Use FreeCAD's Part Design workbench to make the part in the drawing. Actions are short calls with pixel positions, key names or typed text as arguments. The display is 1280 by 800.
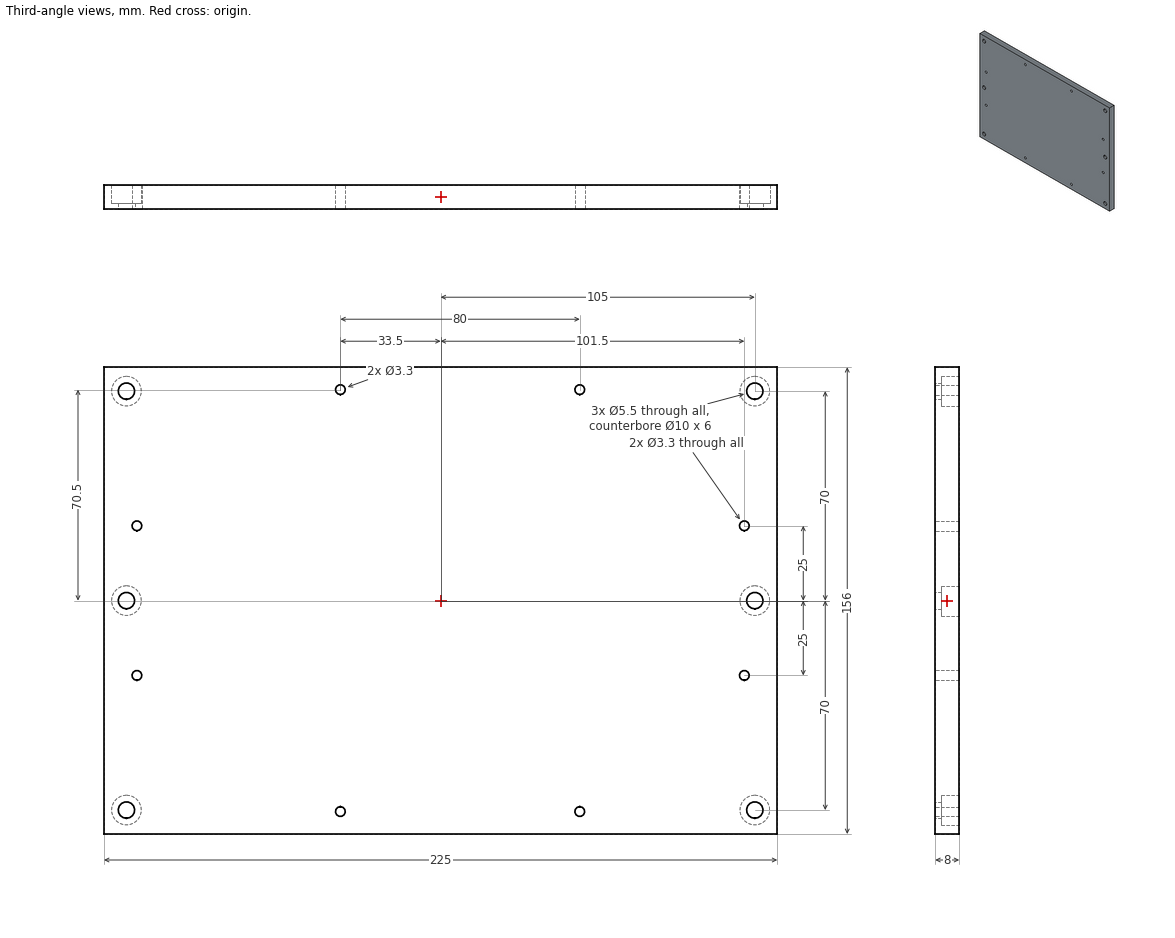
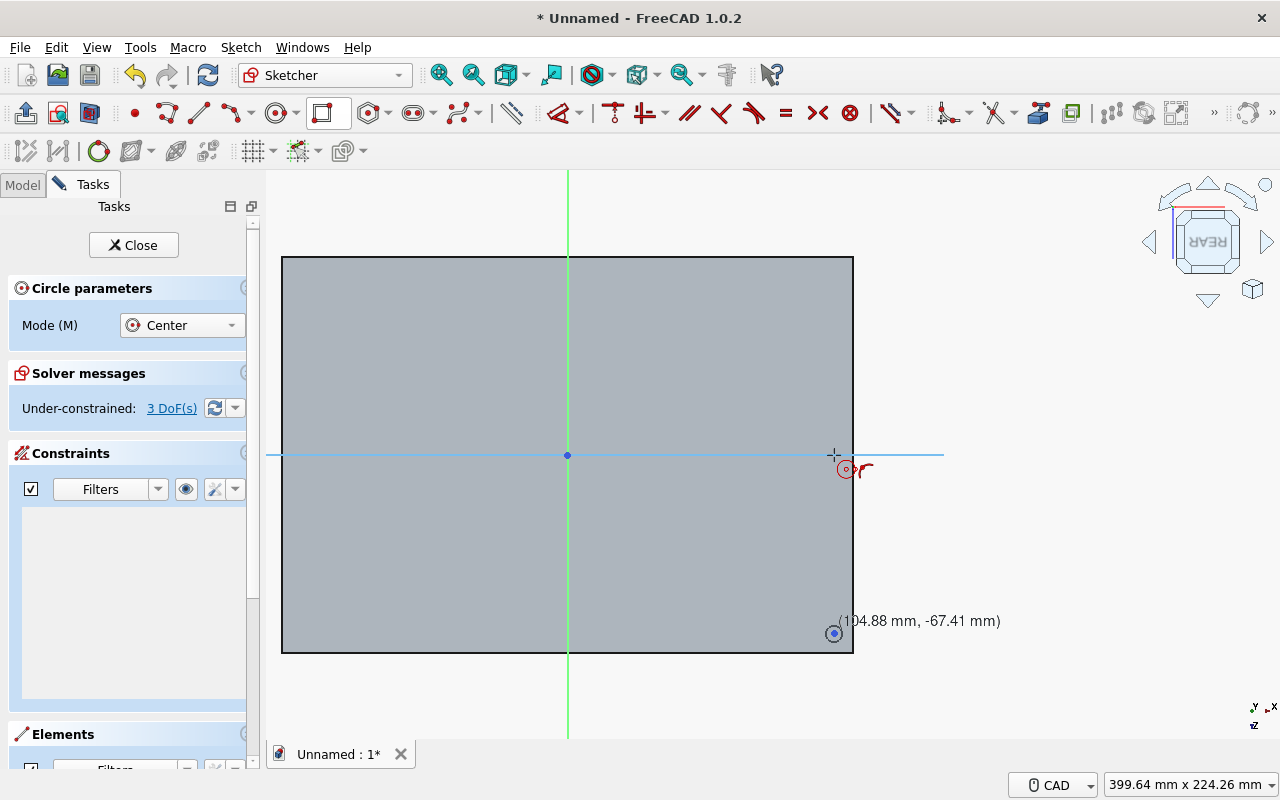
click(834, 455)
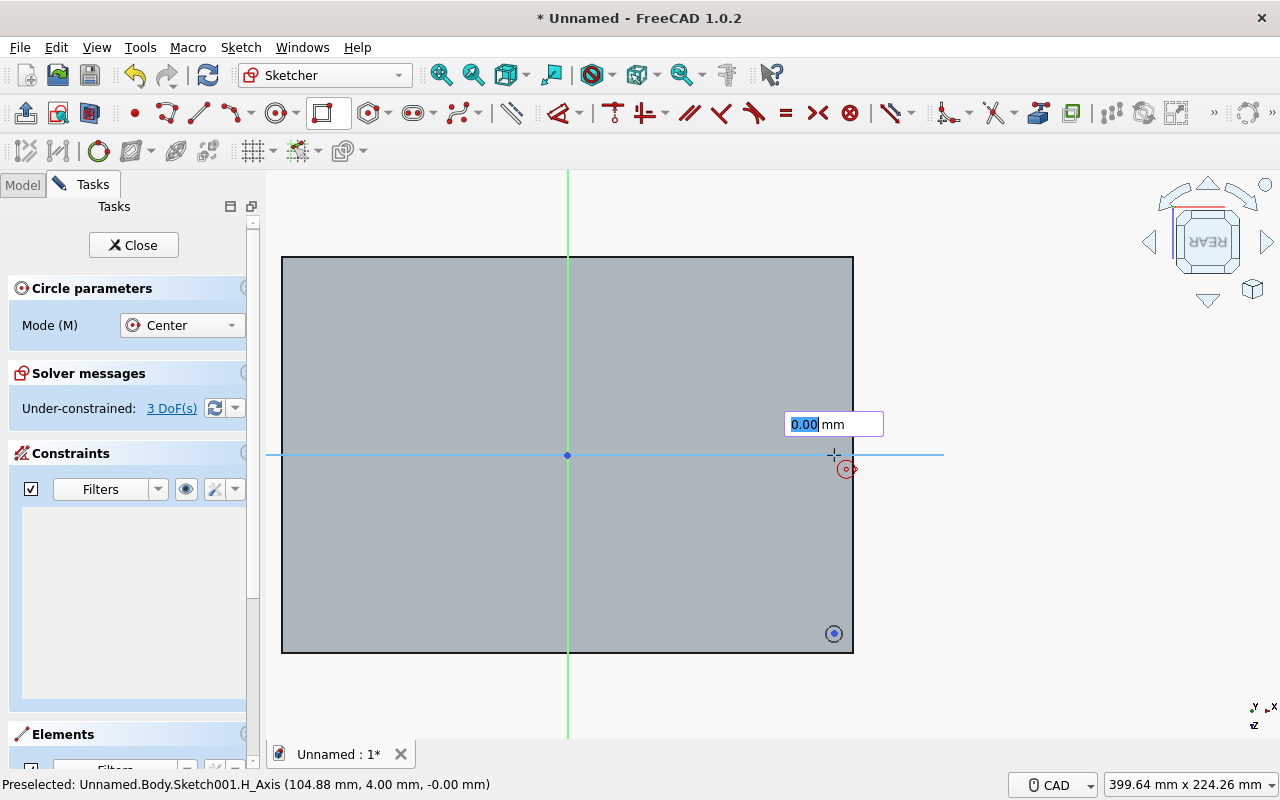
scroll(837, 448, up, 5)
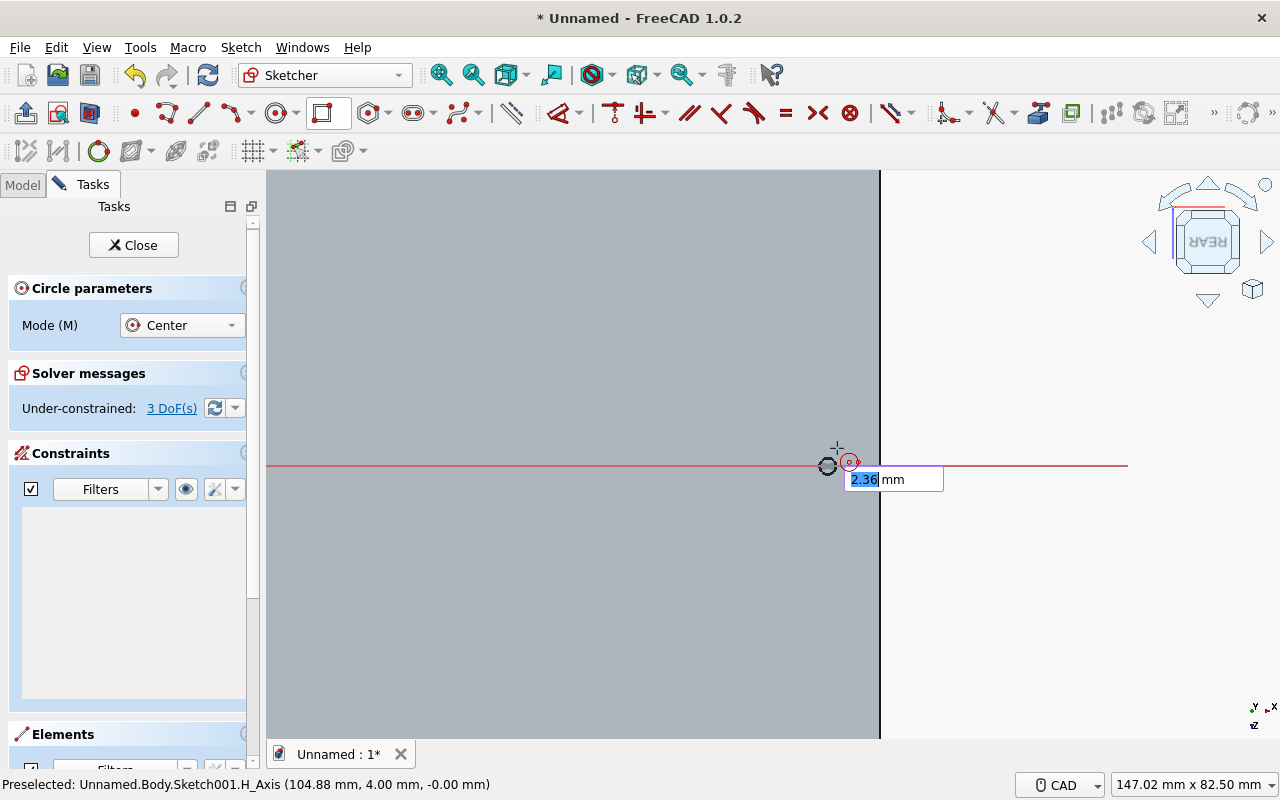
click(835, 448)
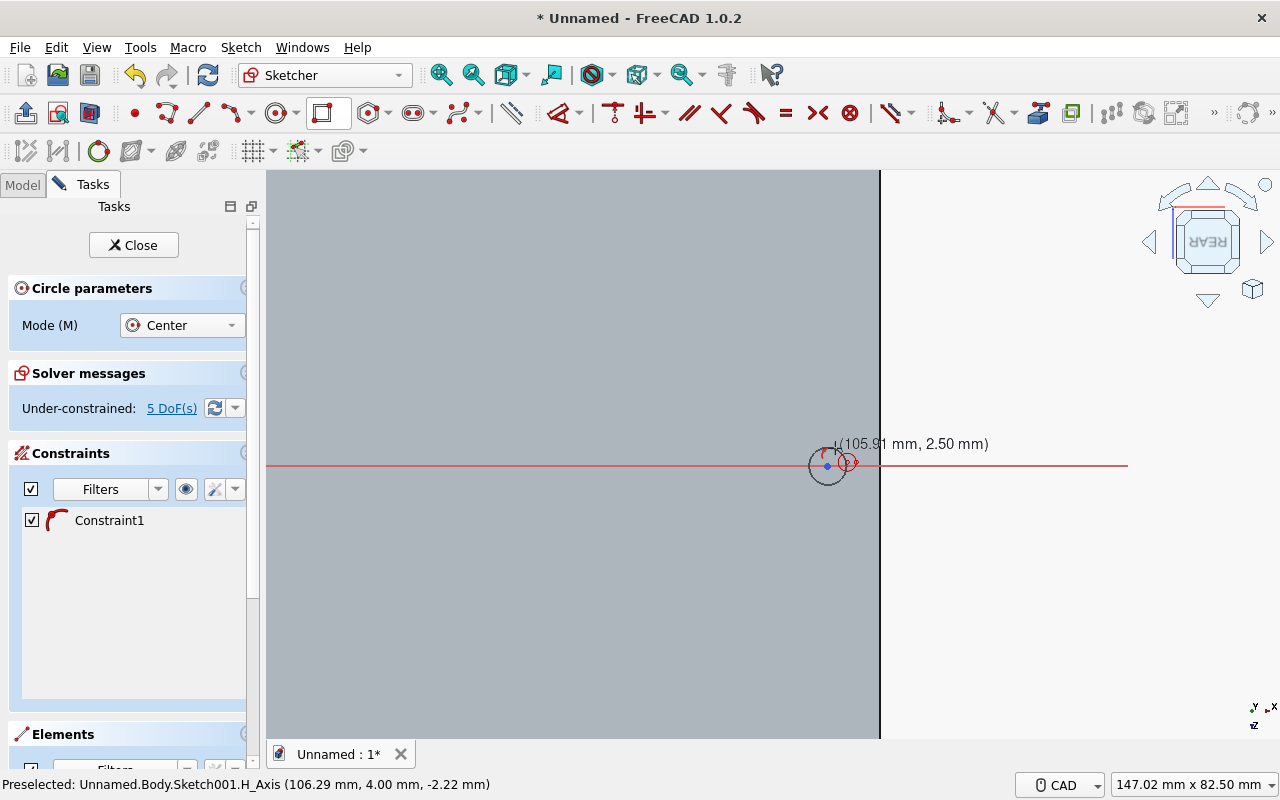
scroll(837, 448, down, 5)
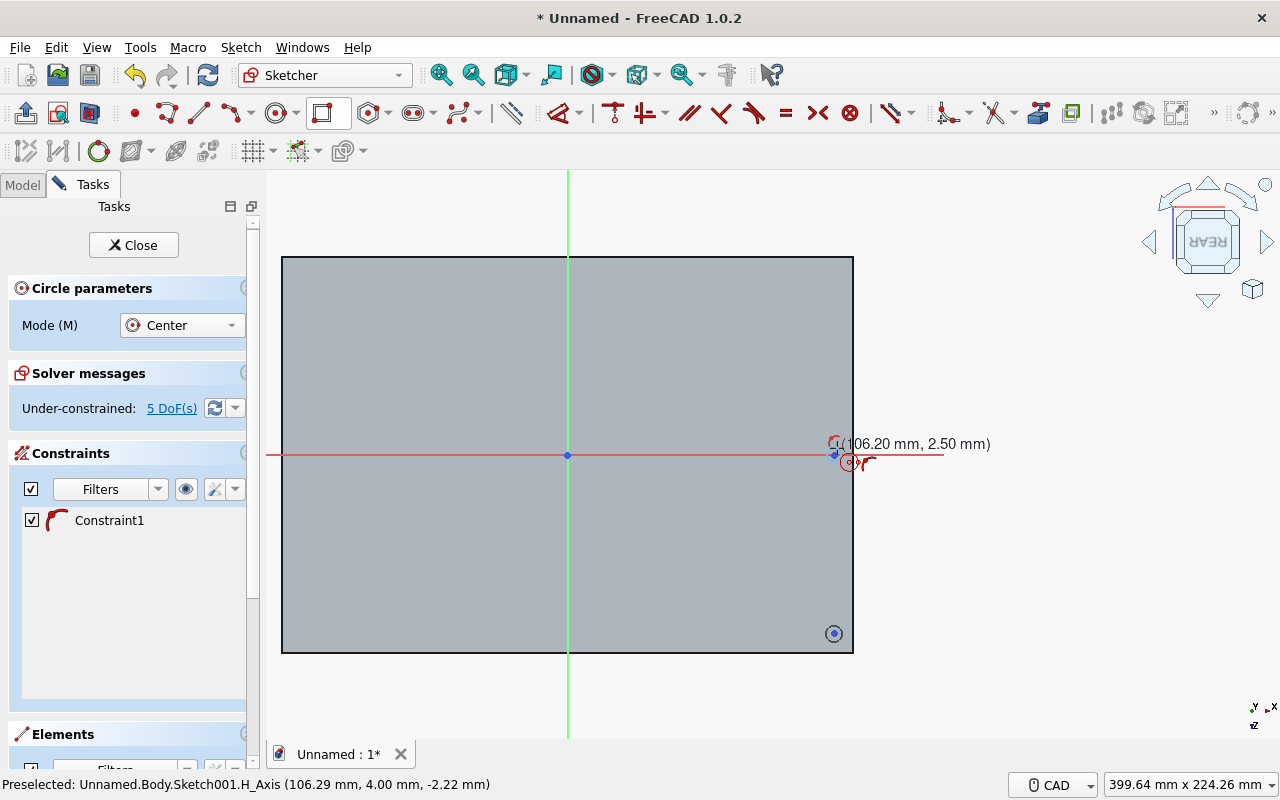
scroll(834, 277, up, 6)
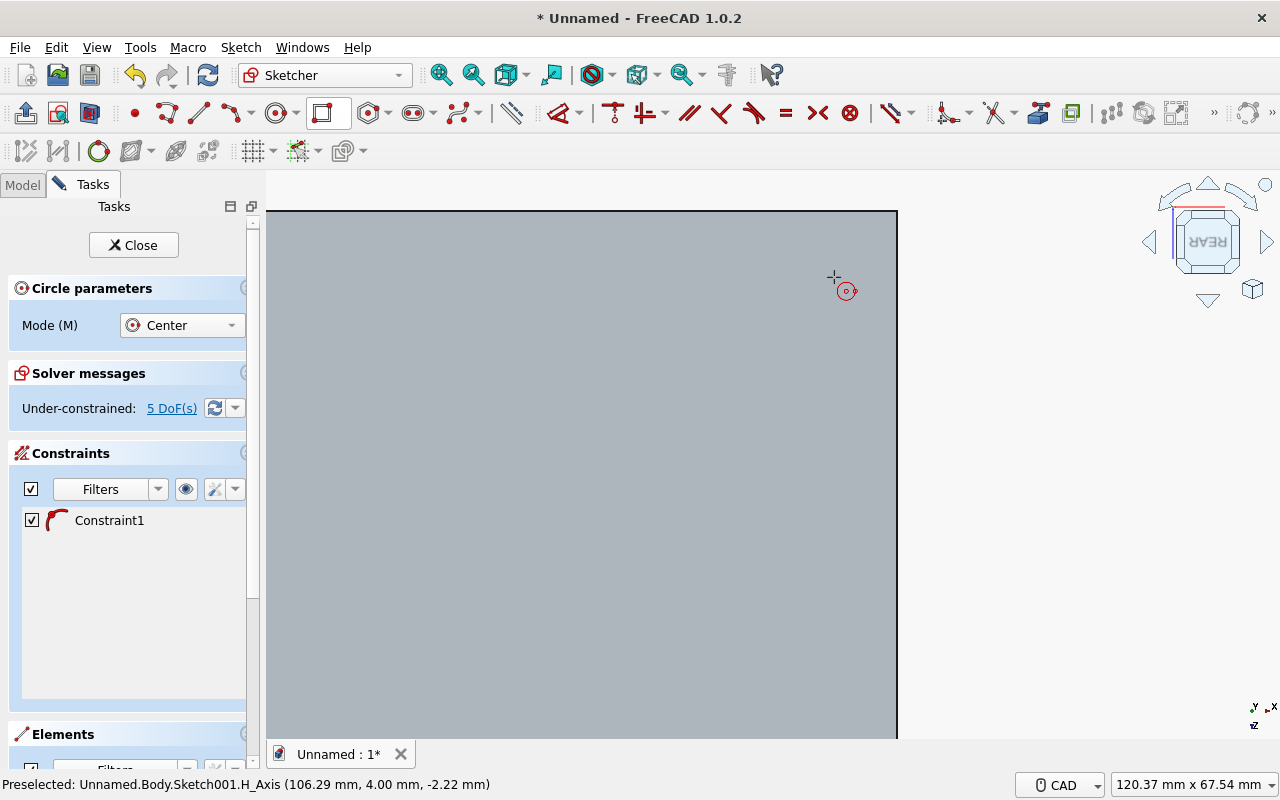
scroll(834, 276, down, 6)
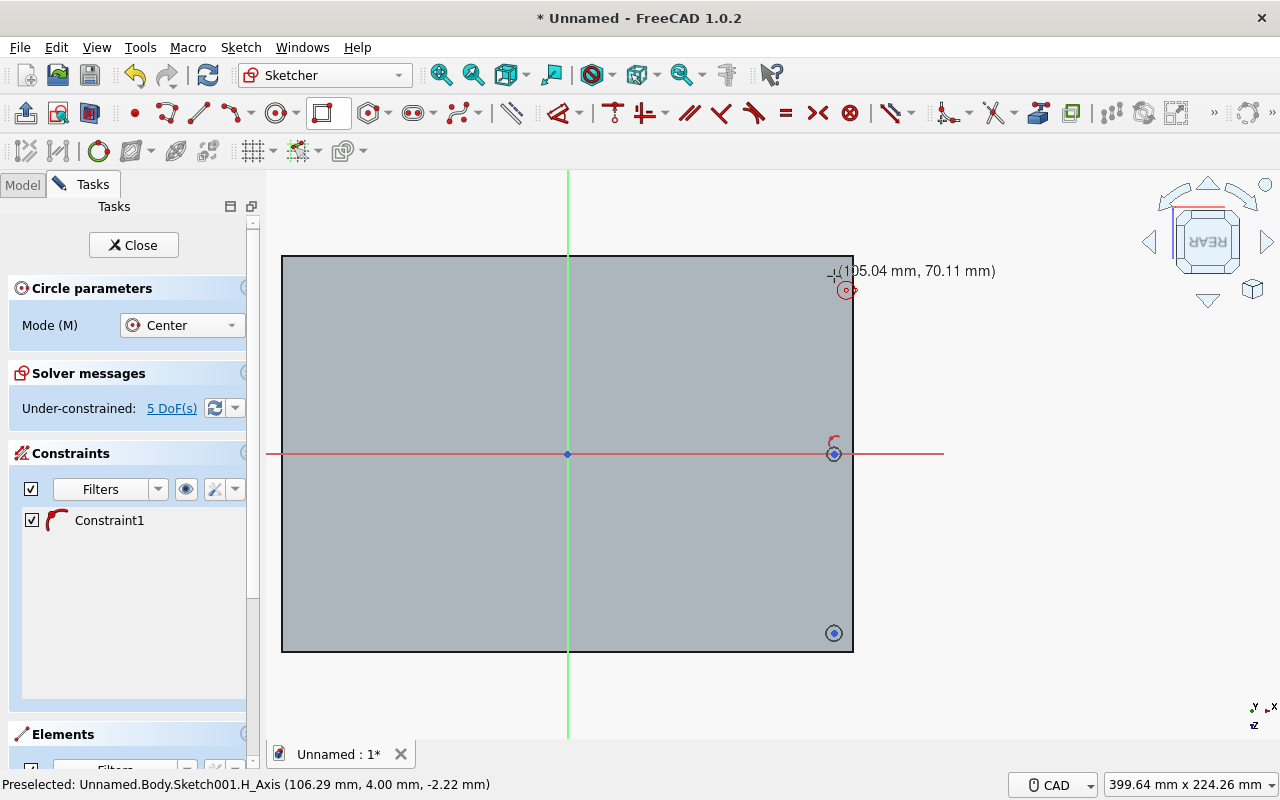
click(834, 277)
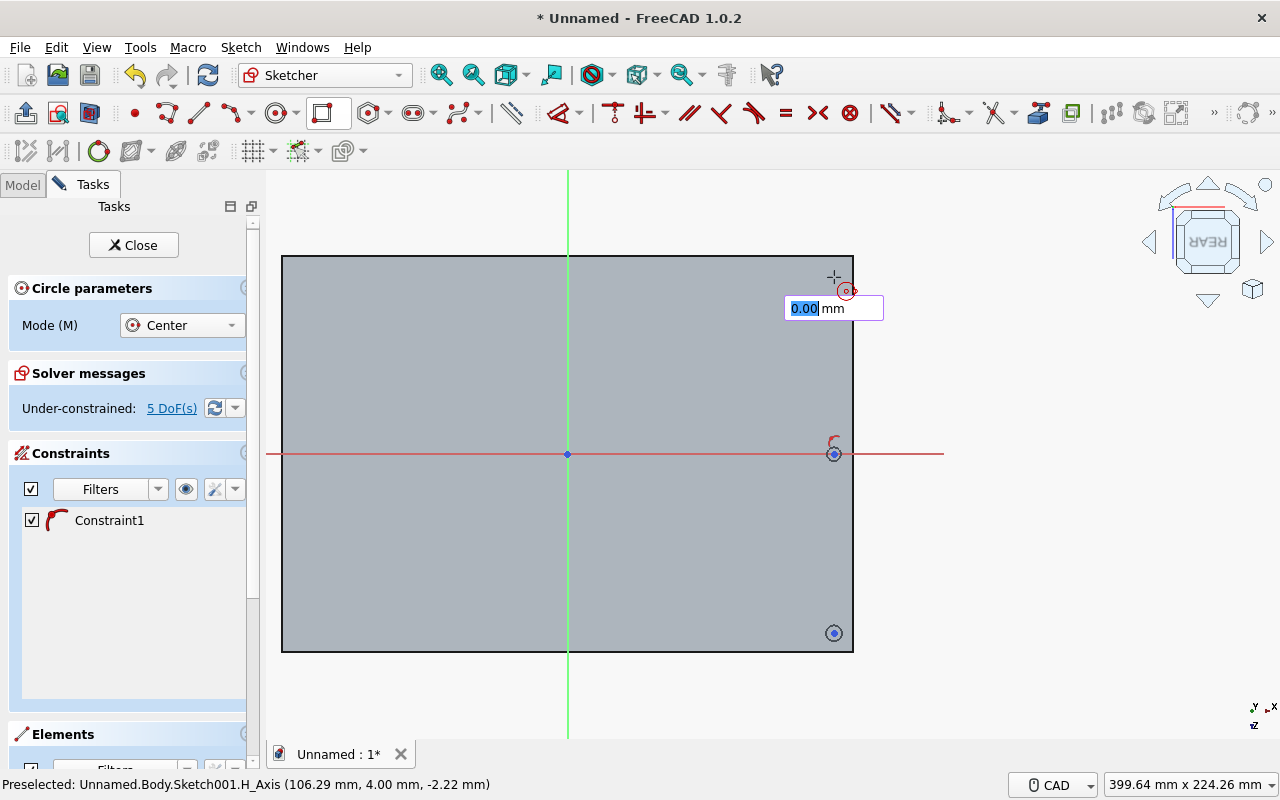
scroll(839, 272, up, 5)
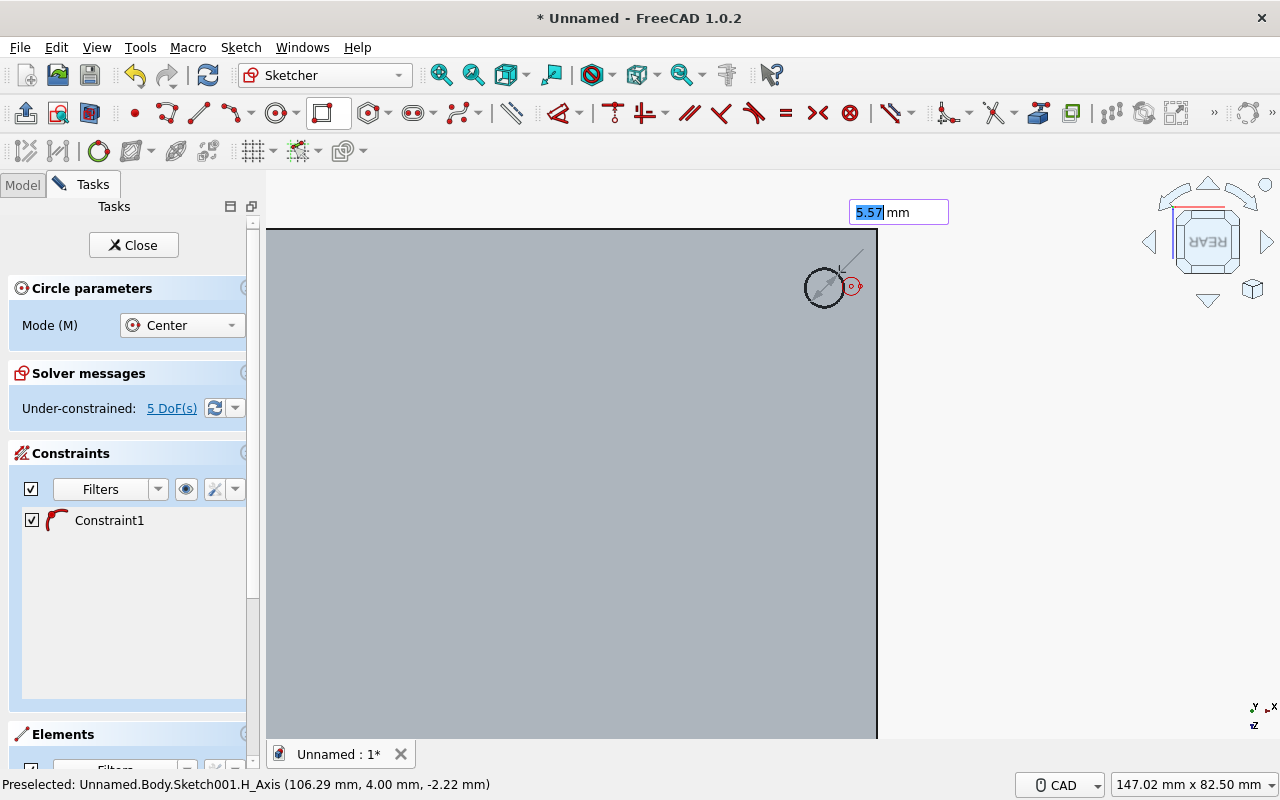
click(839, 271)
key(Escape)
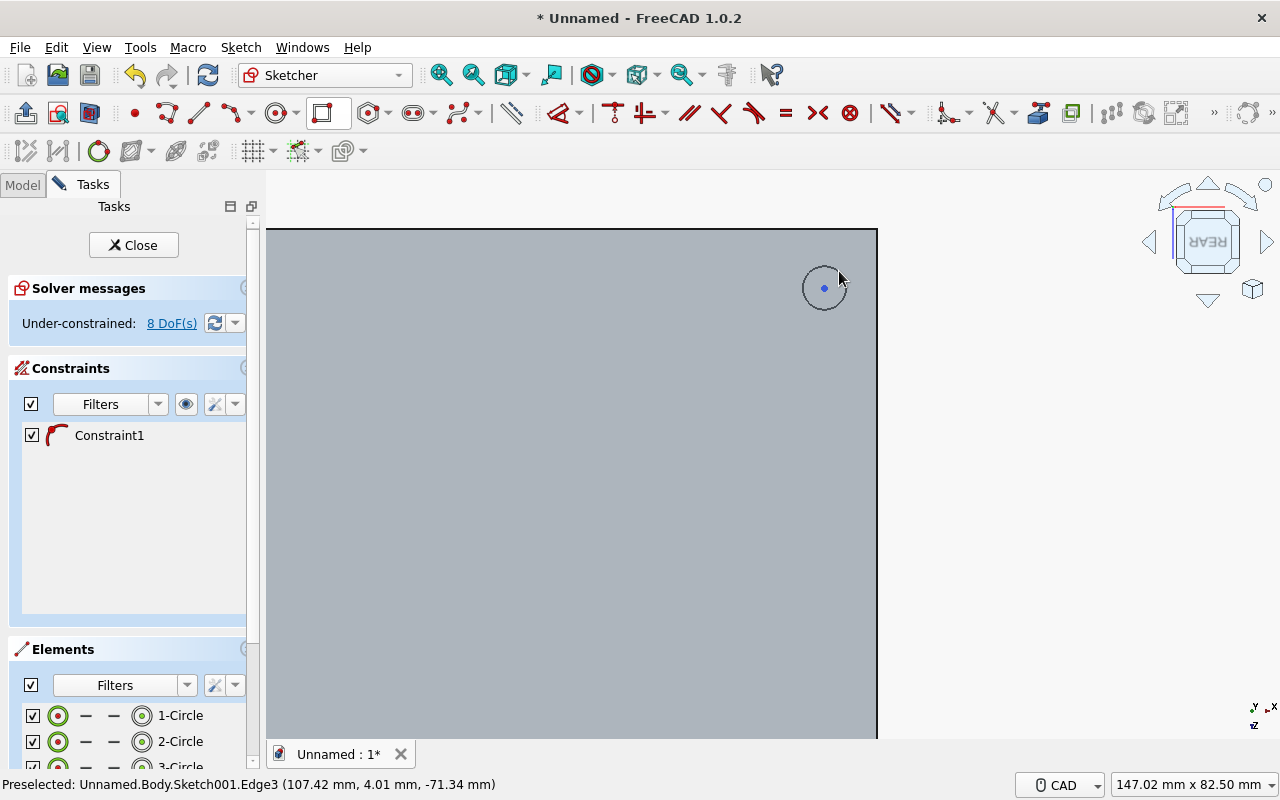
scroll(839, 272, down, 5)